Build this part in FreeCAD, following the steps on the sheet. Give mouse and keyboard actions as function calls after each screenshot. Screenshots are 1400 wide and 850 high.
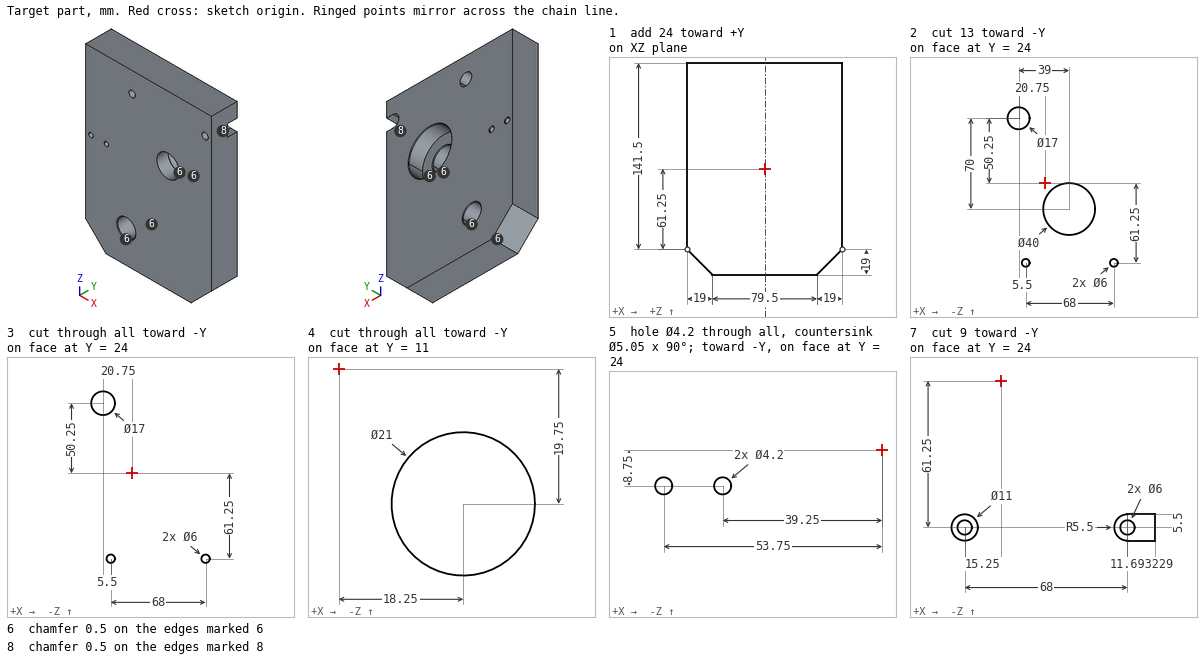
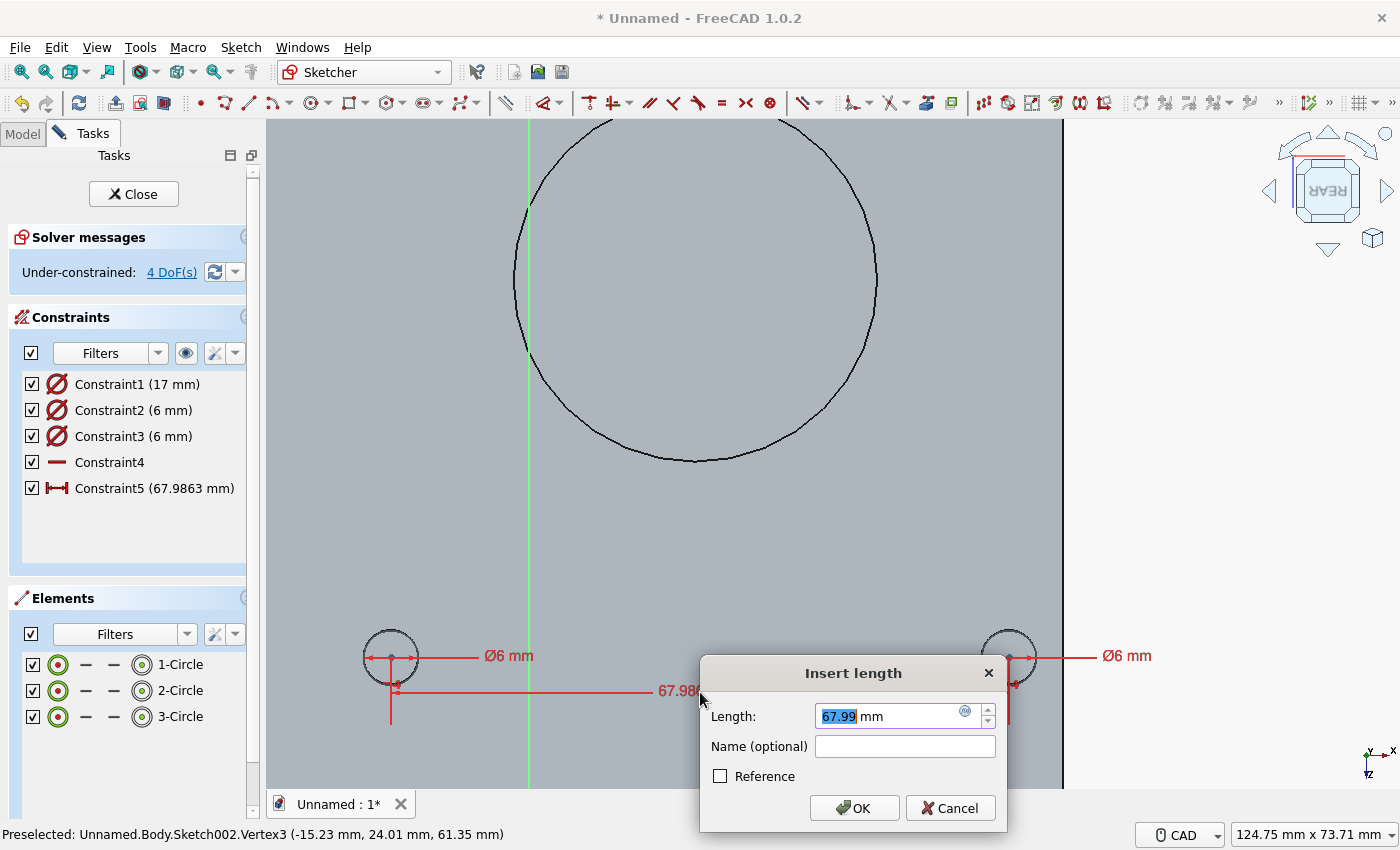
text(68)
key(Return)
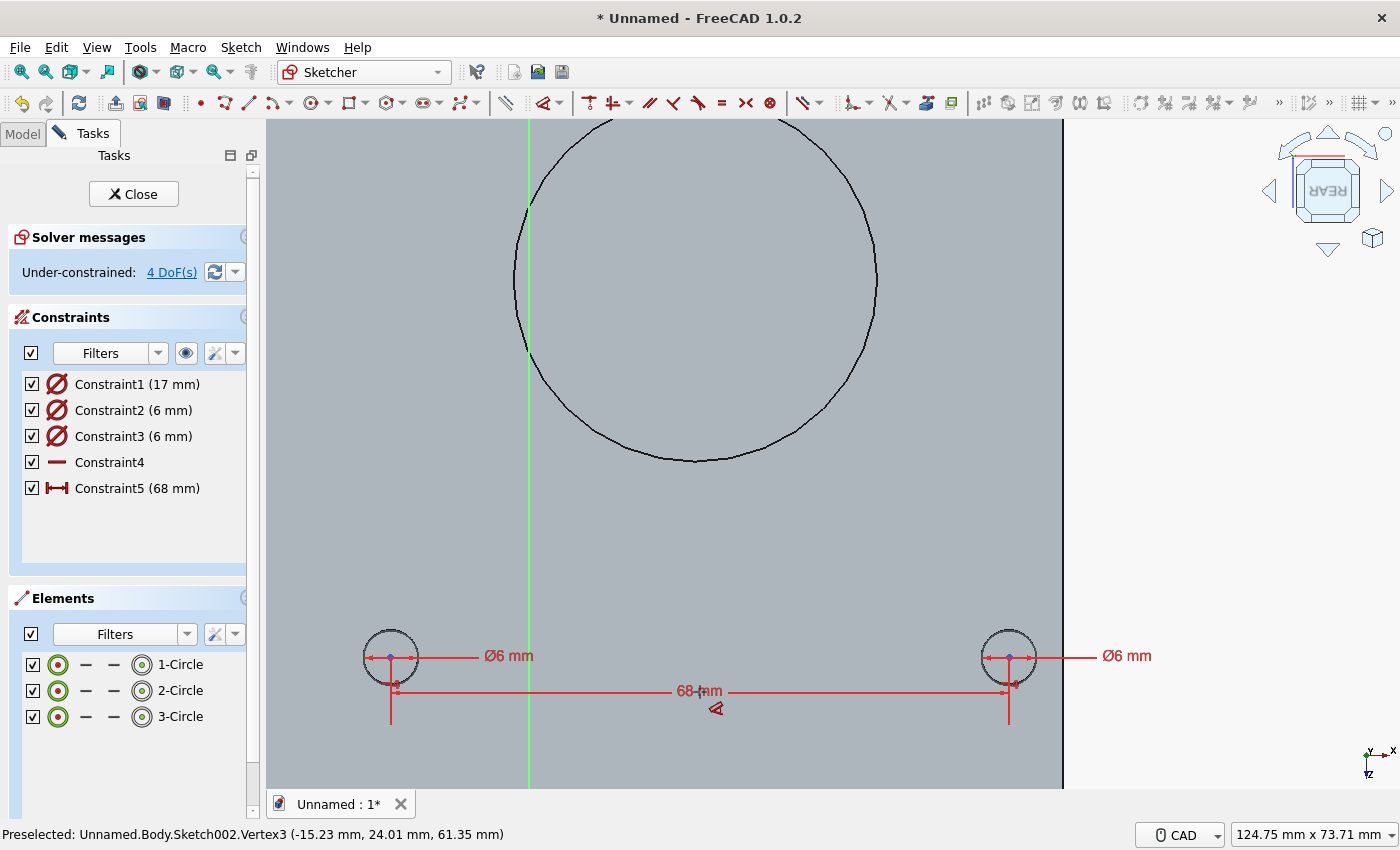
scroll(831, 645, down, 5)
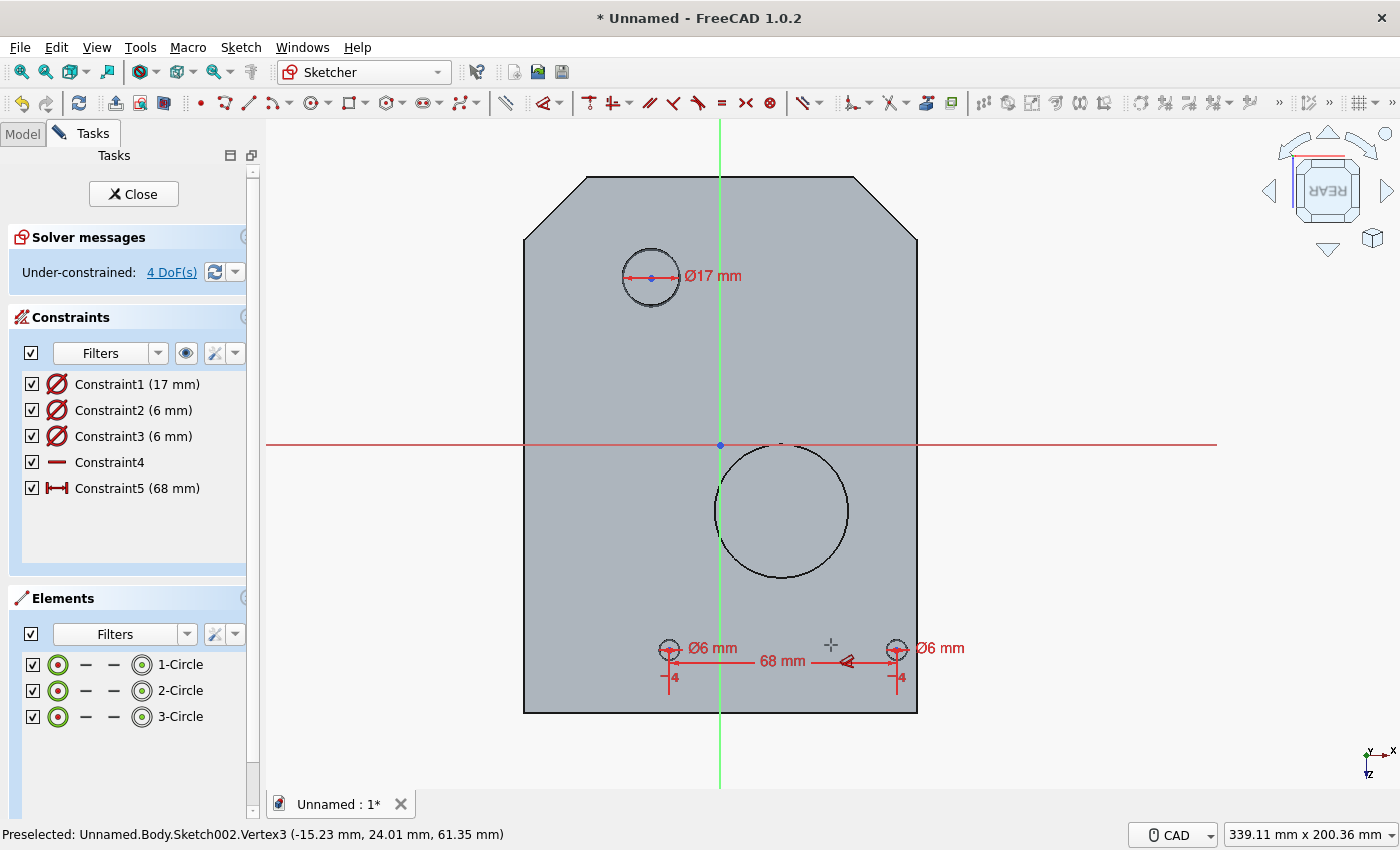
scroll(651, 278, up, 4)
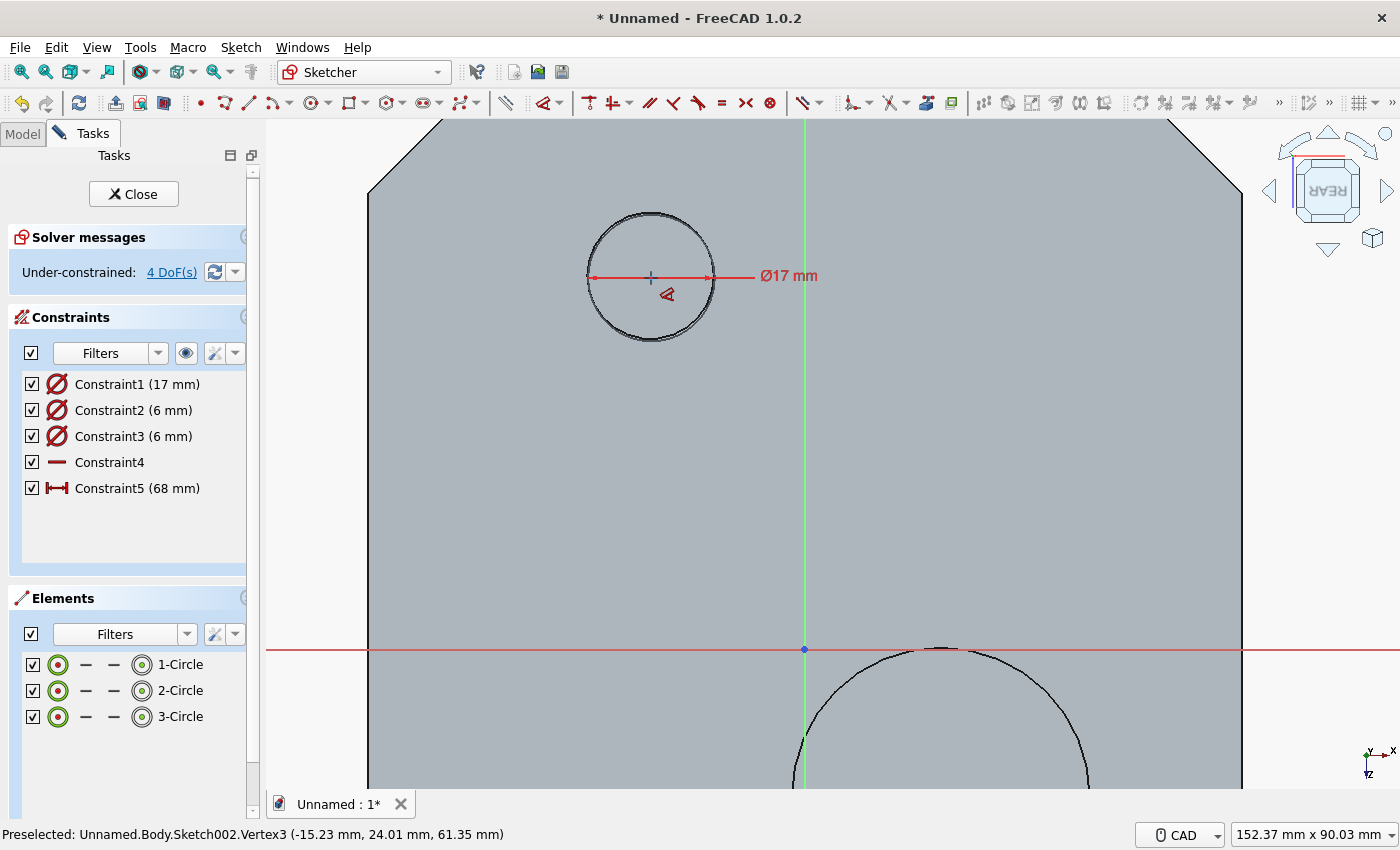
click(651, 278)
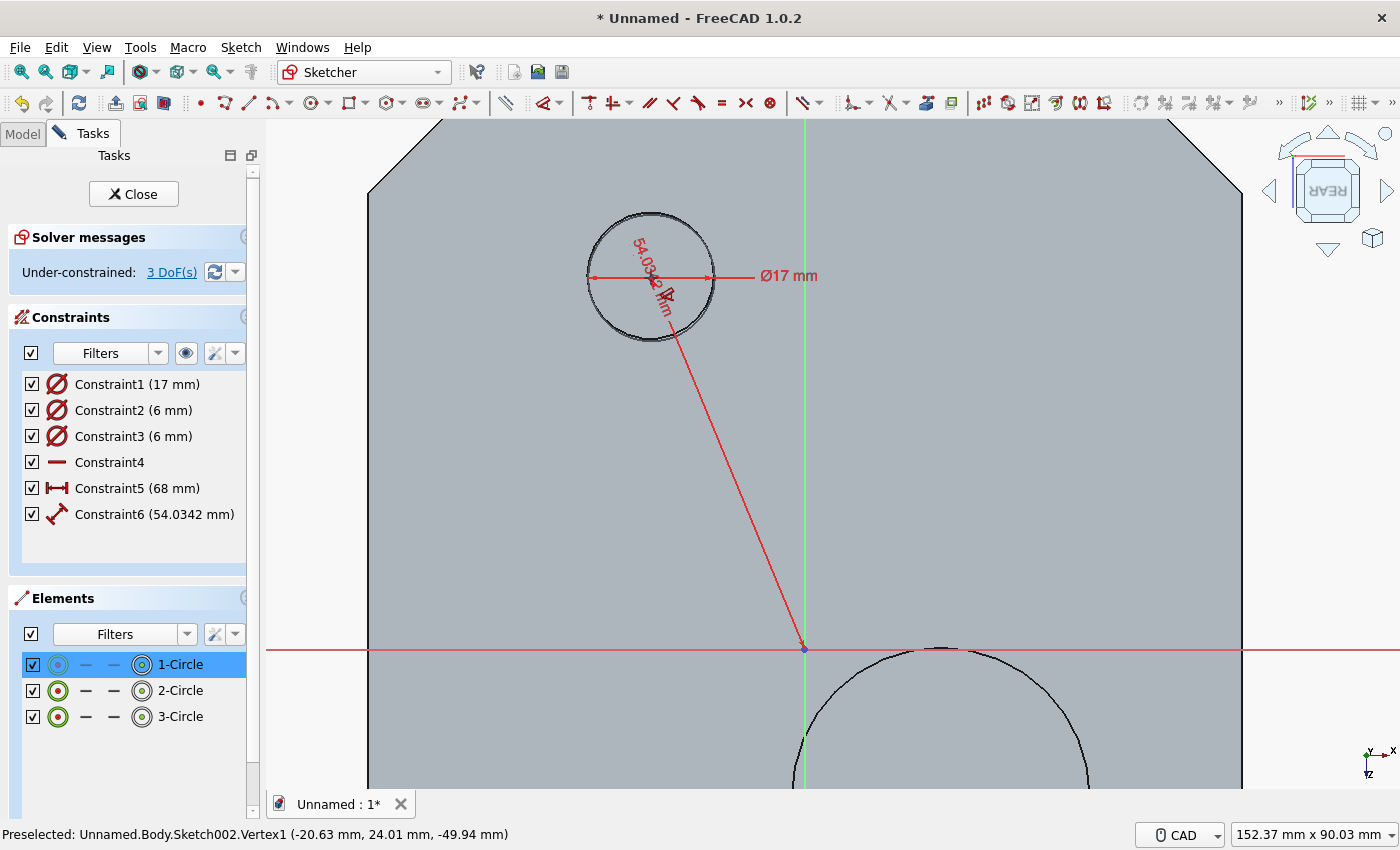
scroll(651, 278, down, 4)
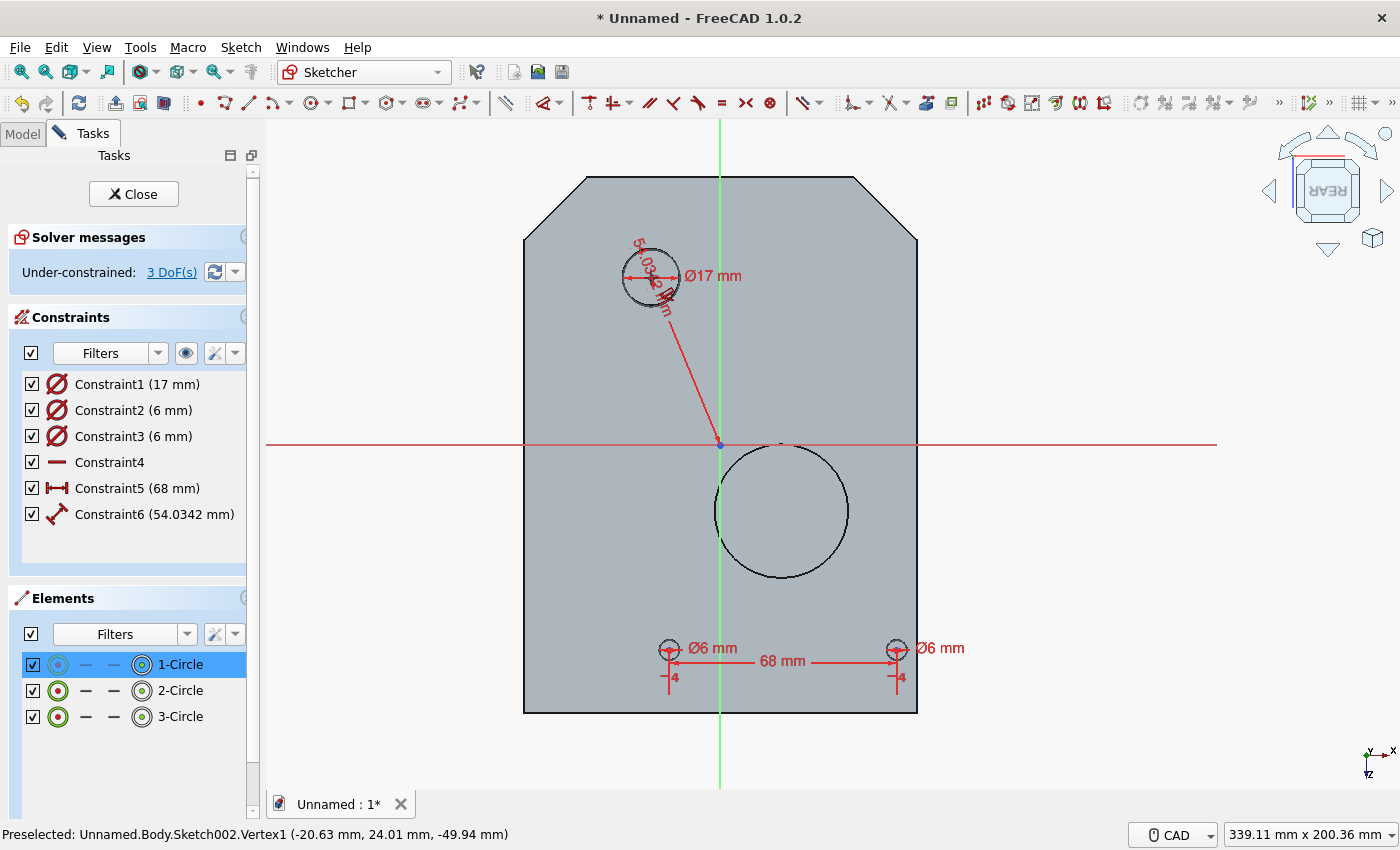
scroll(669, 650, up, 4)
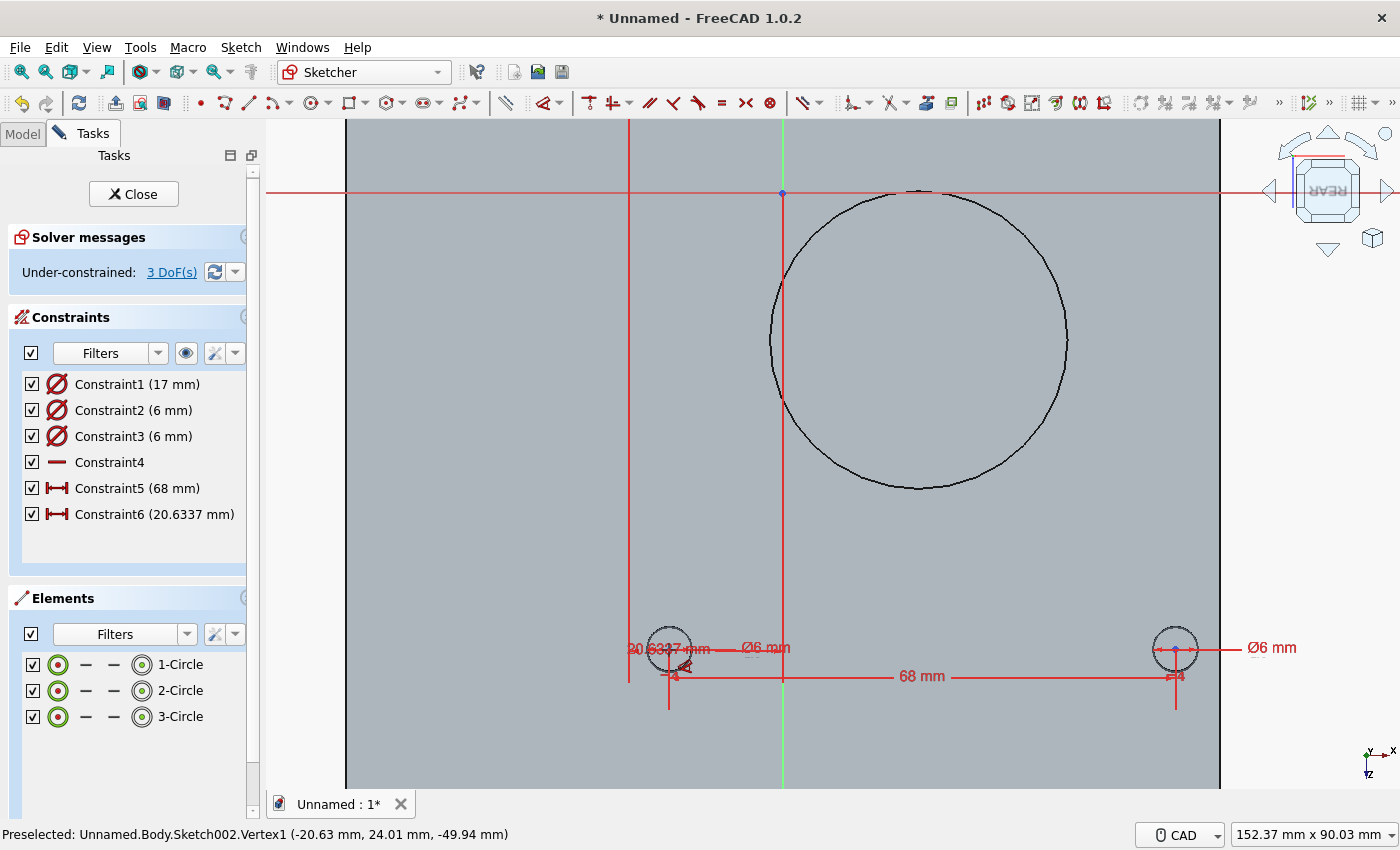
click(669, 650)
click(649, 684)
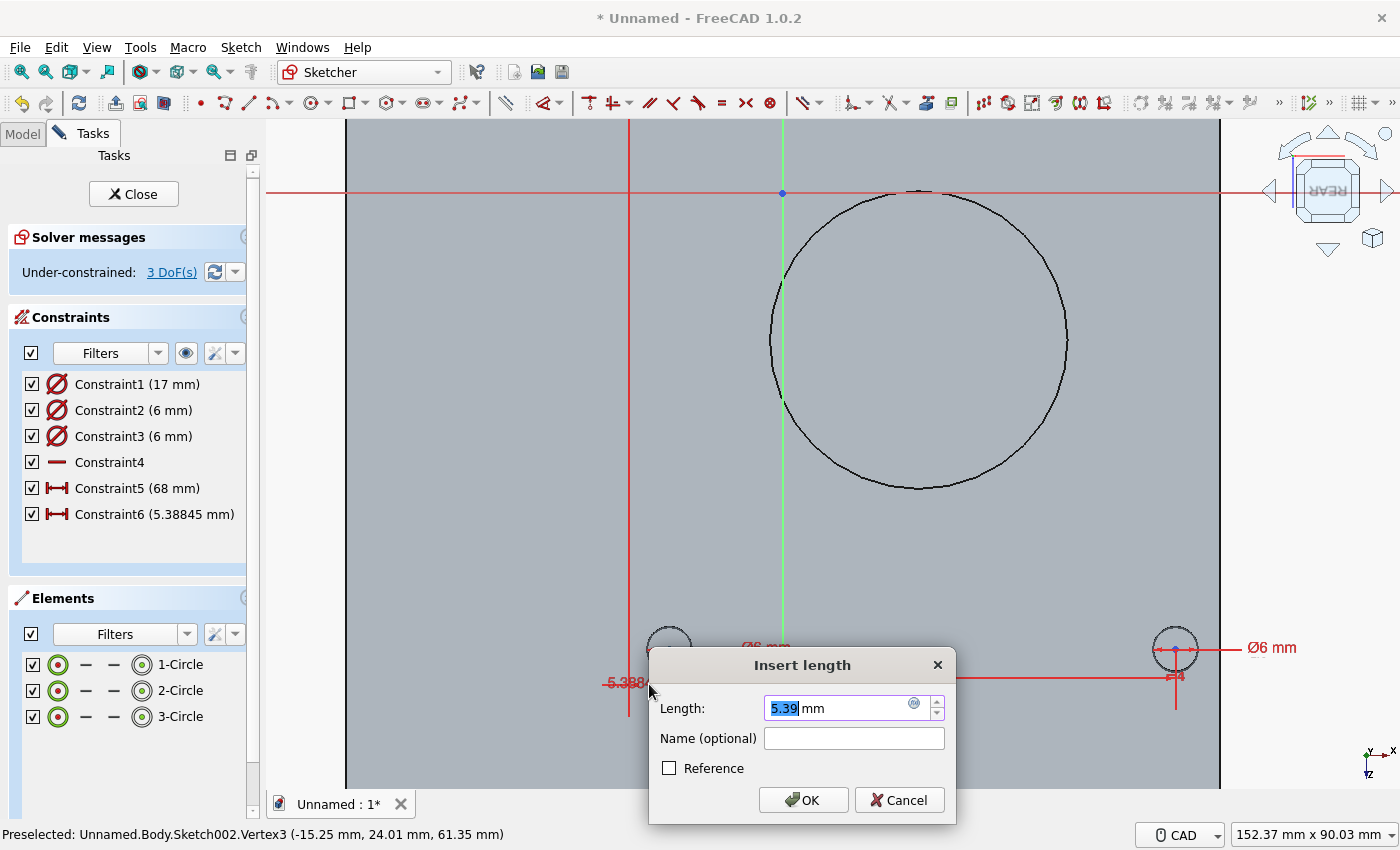
text(5.5)
key(Return)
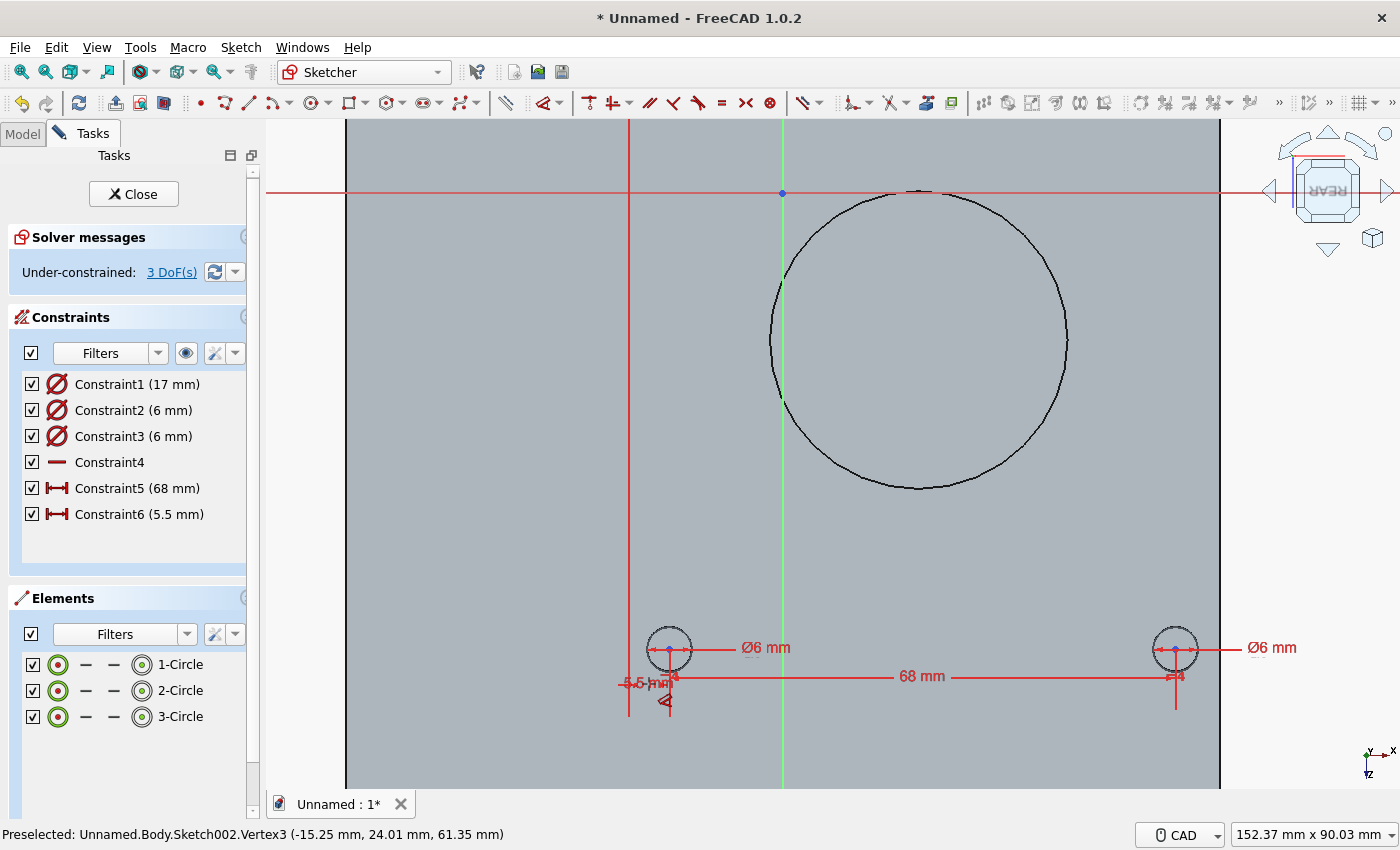
scroll(669, 650, down, 4)